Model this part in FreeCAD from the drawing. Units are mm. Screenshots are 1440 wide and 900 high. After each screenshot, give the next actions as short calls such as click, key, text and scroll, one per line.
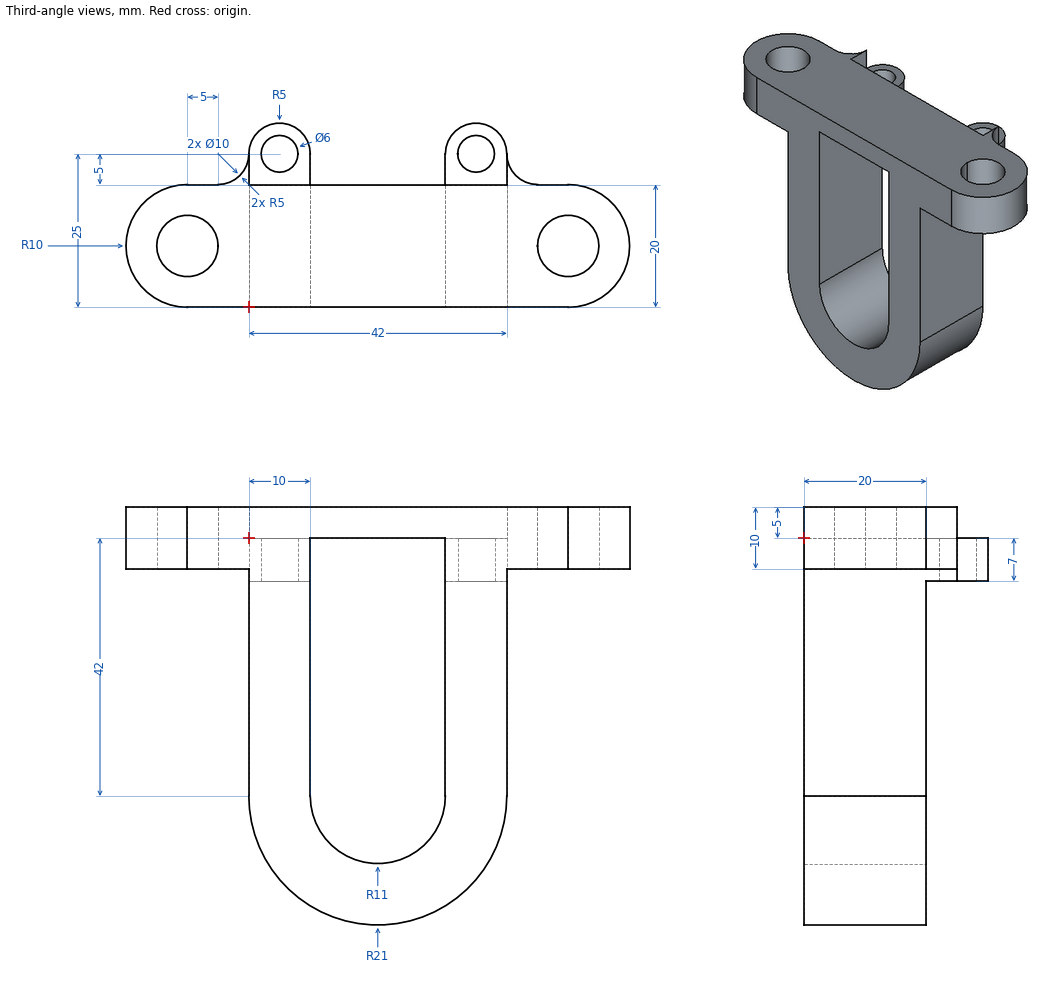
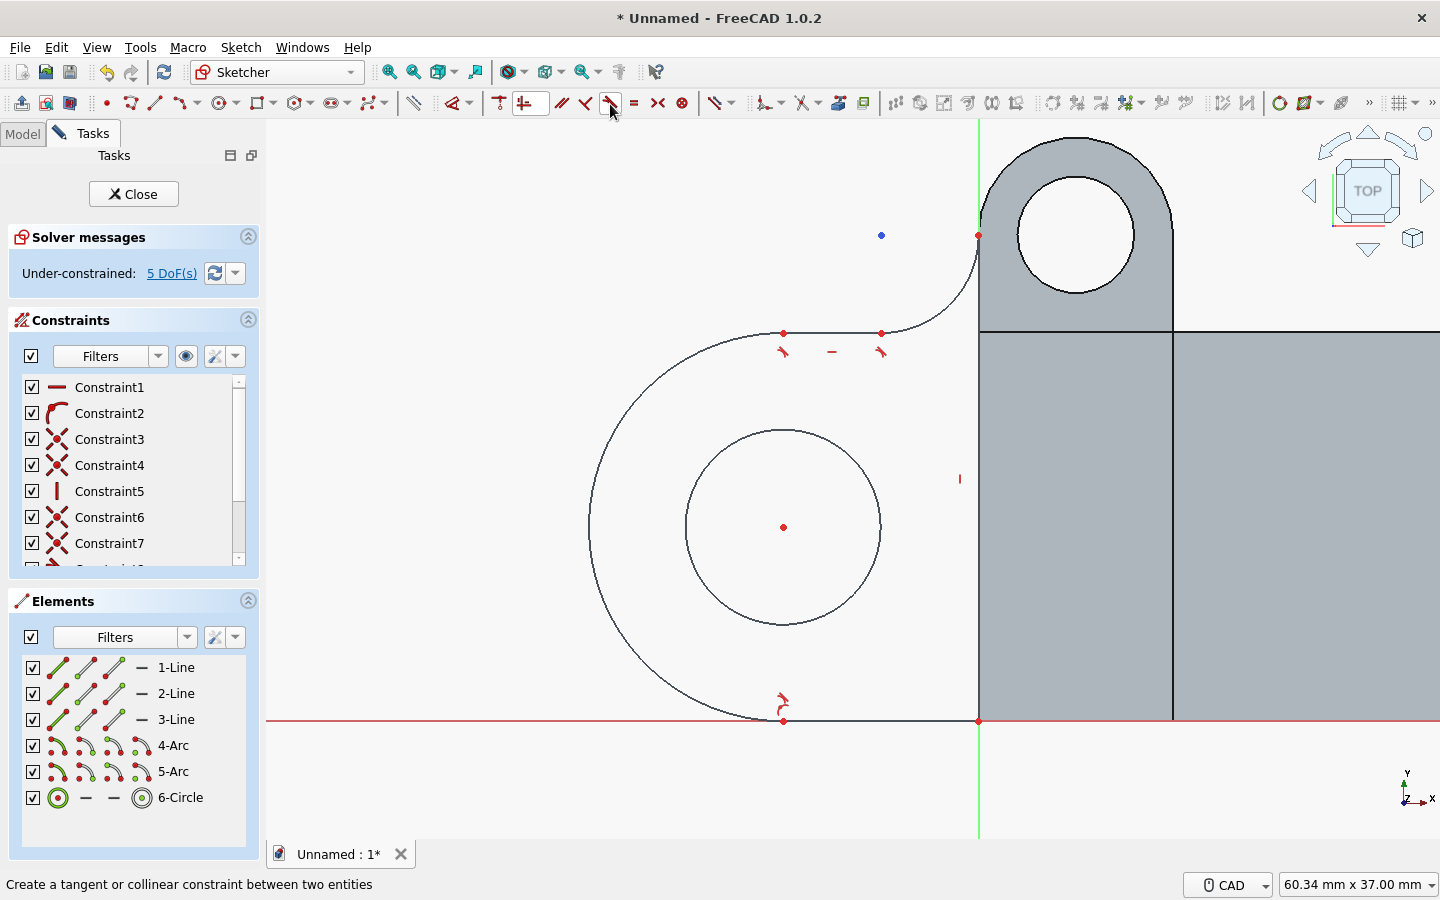
click(979, 576)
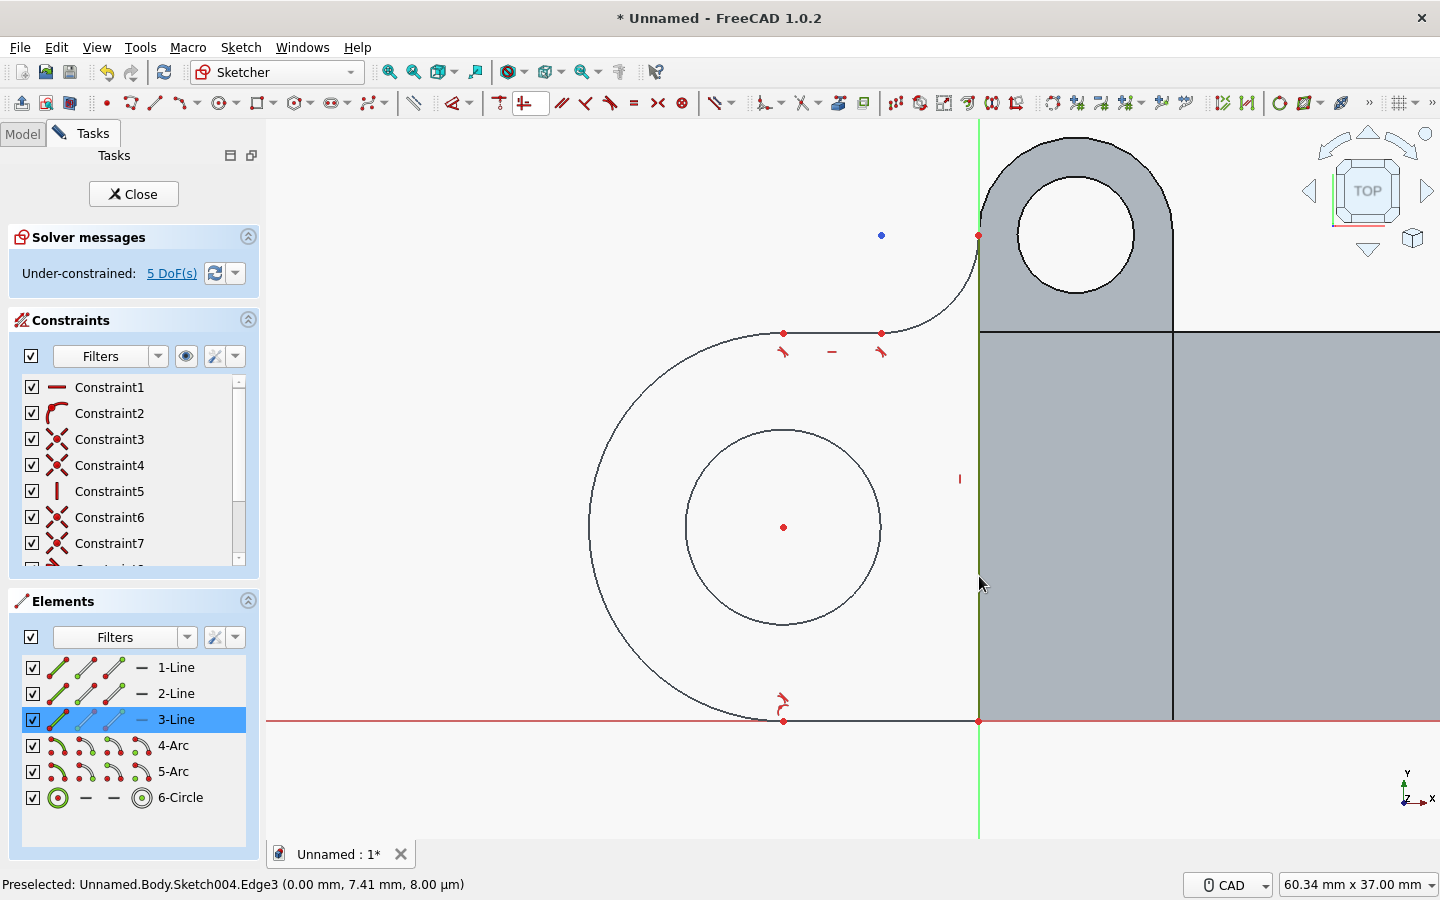
click(925, 322)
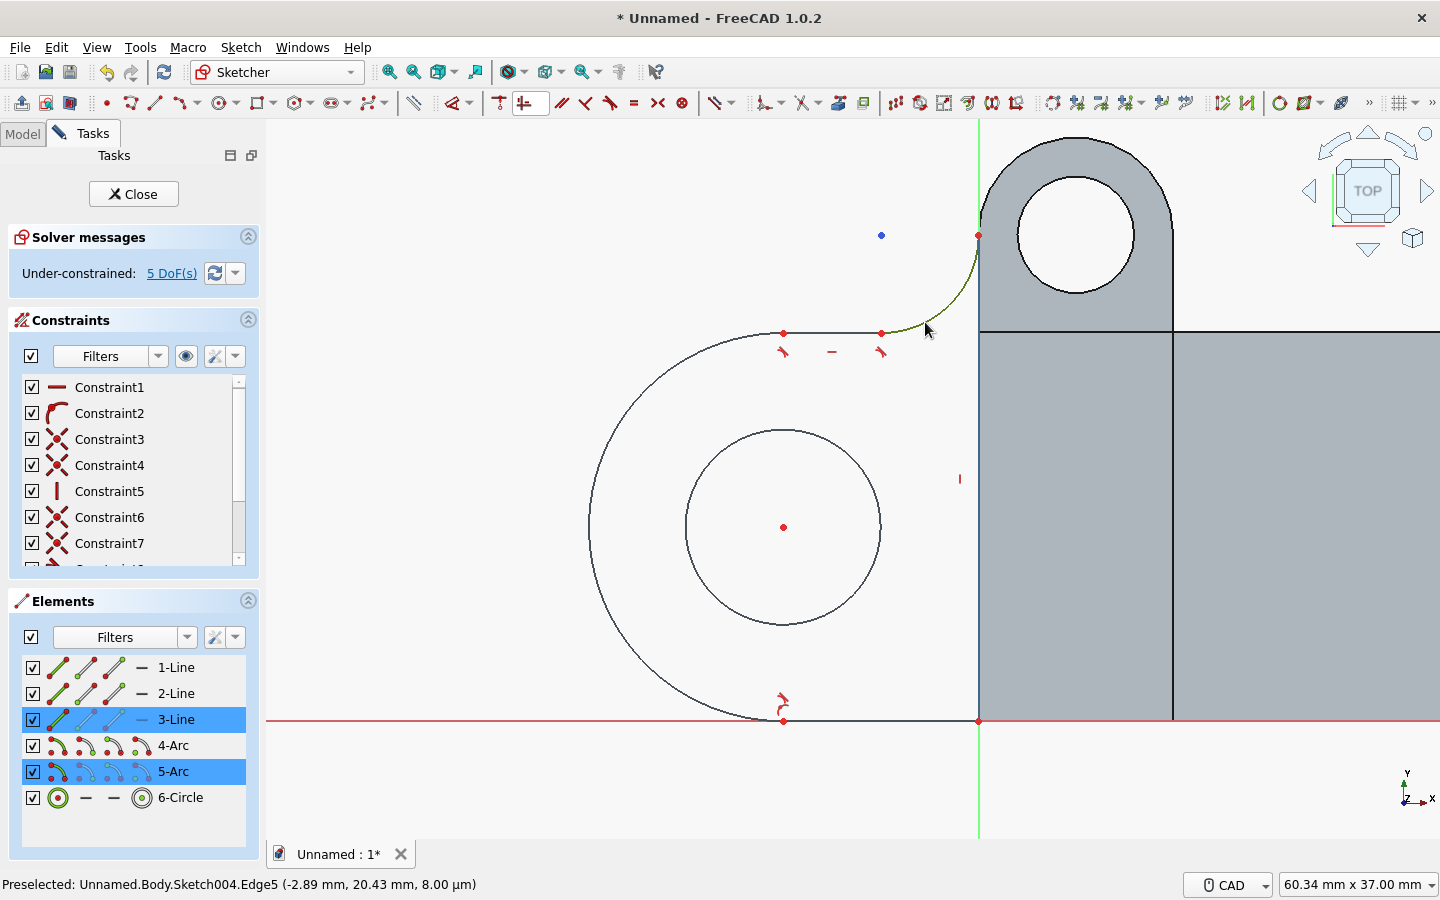
click(610, 104)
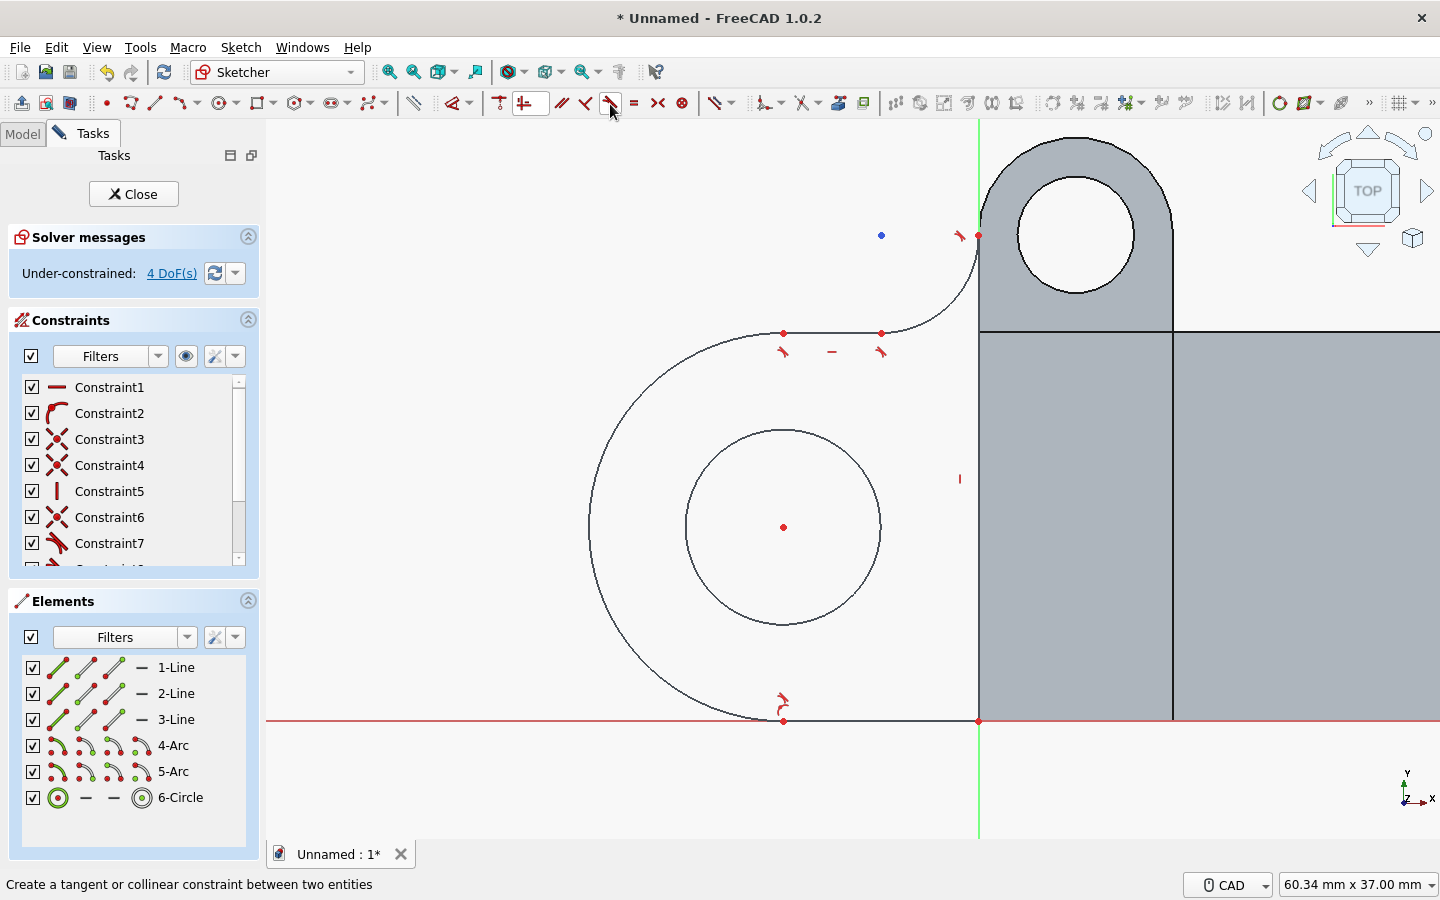
click(452, 104)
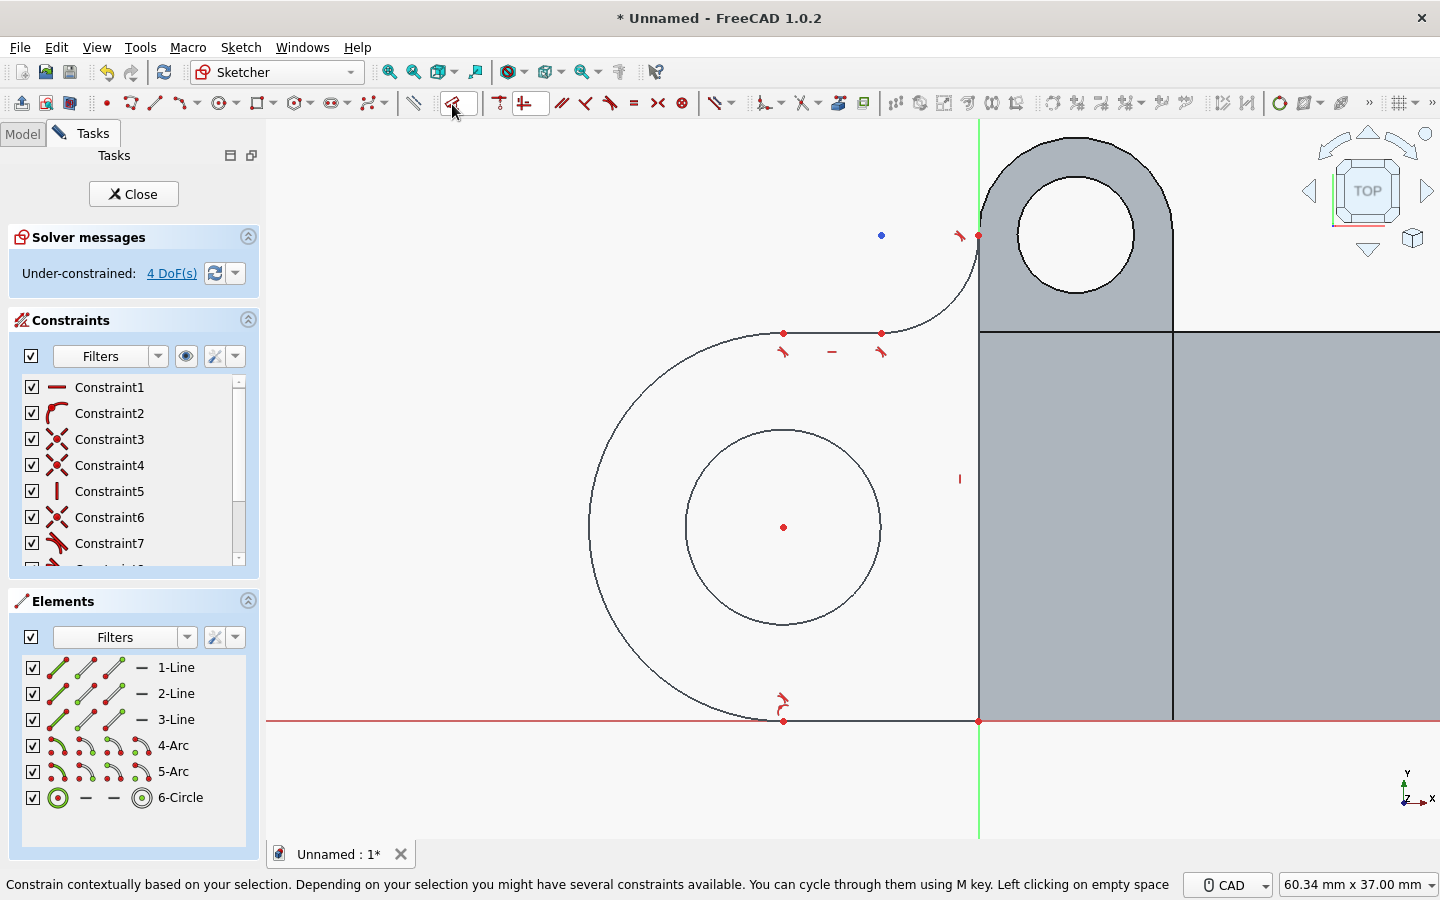
click(626, 413)
click(600, 394)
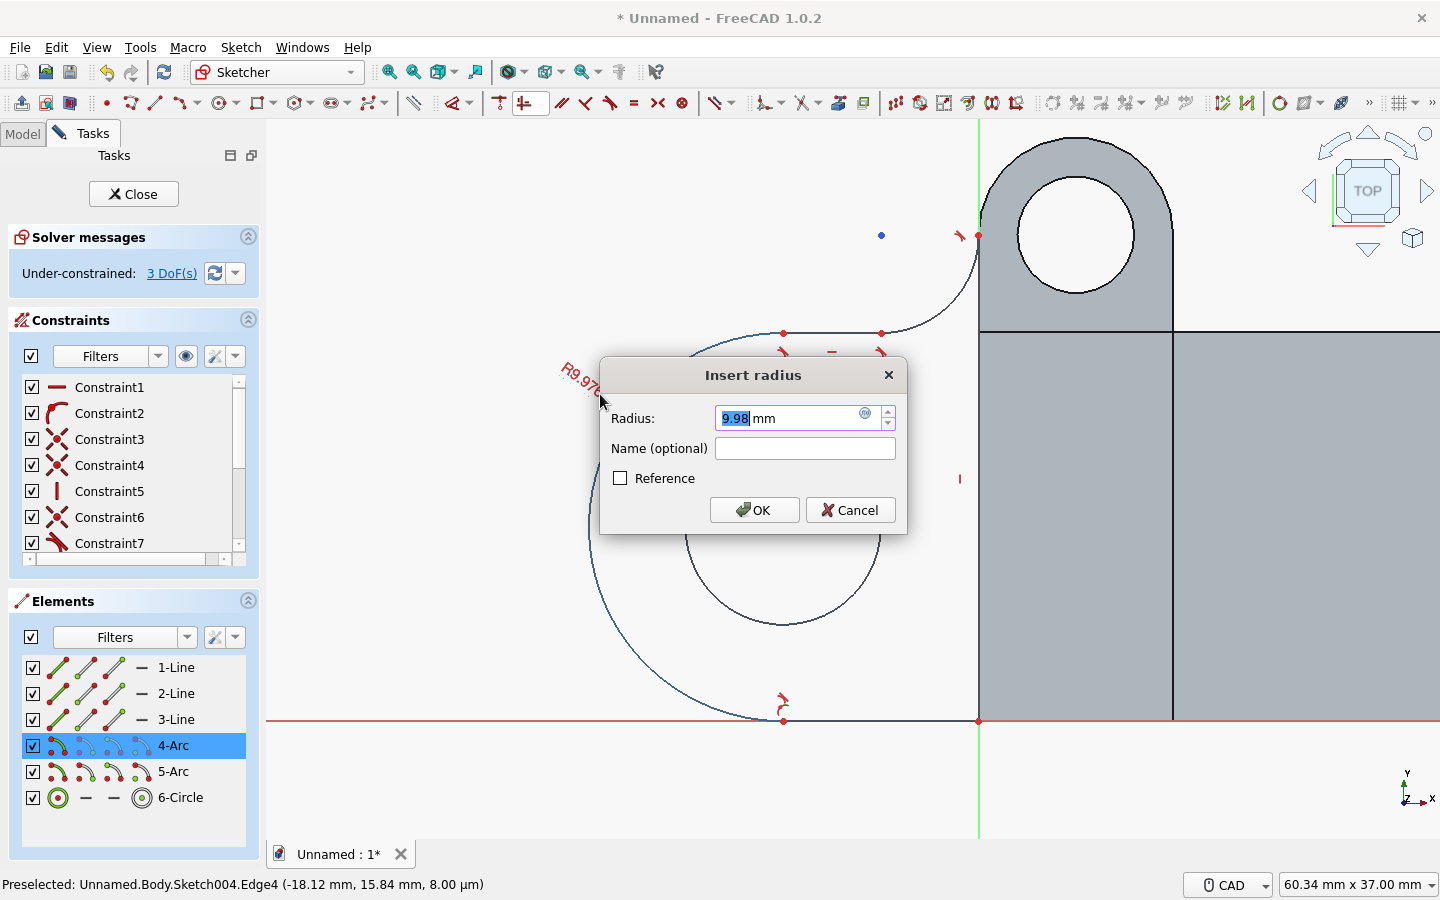
text(10)
key(Return)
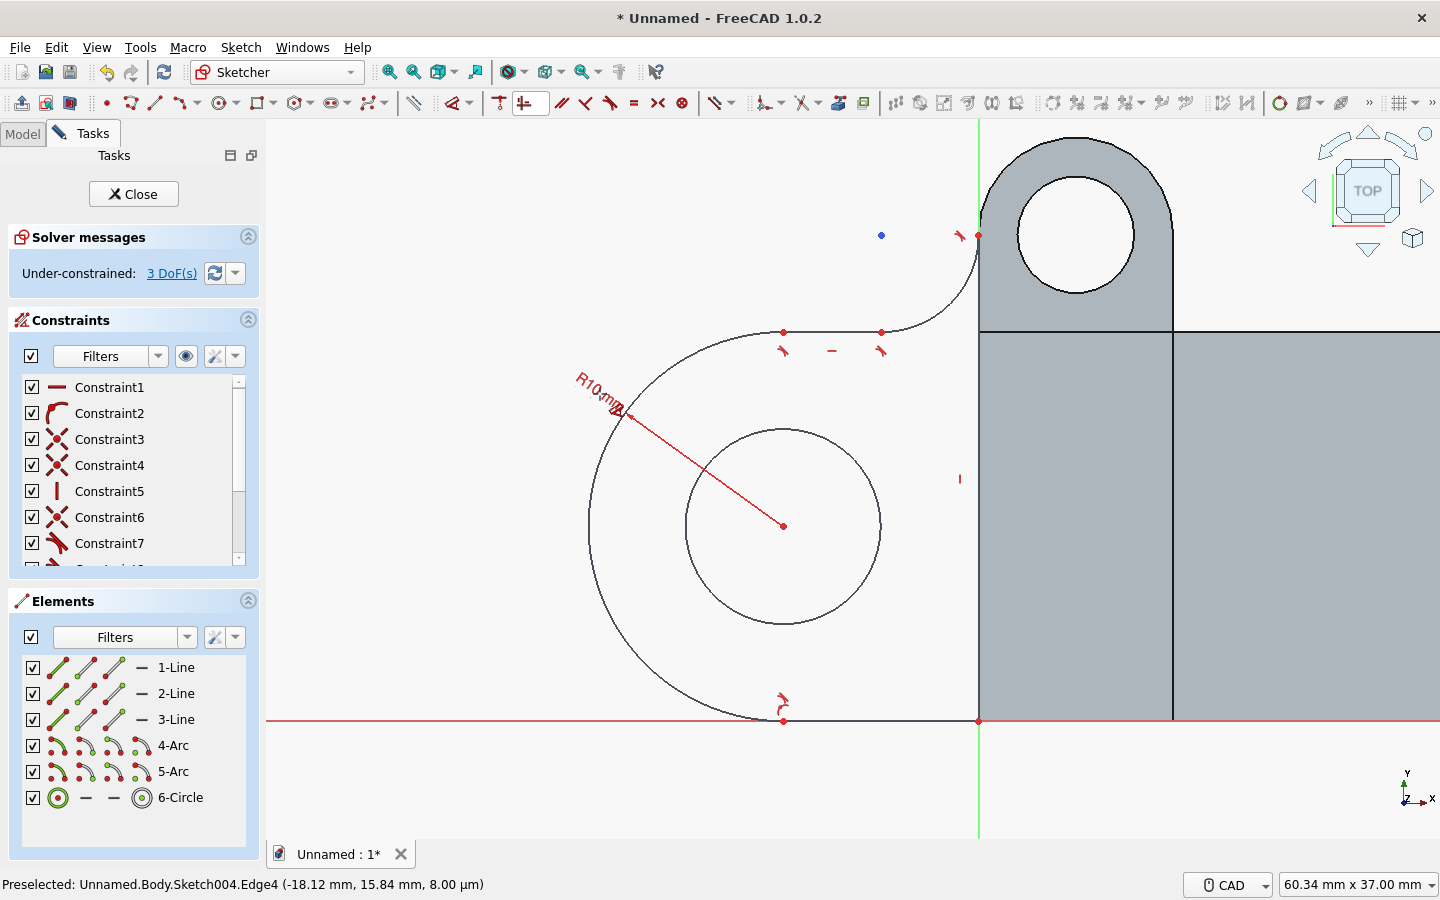
click(926, 322)
click(941, 351)